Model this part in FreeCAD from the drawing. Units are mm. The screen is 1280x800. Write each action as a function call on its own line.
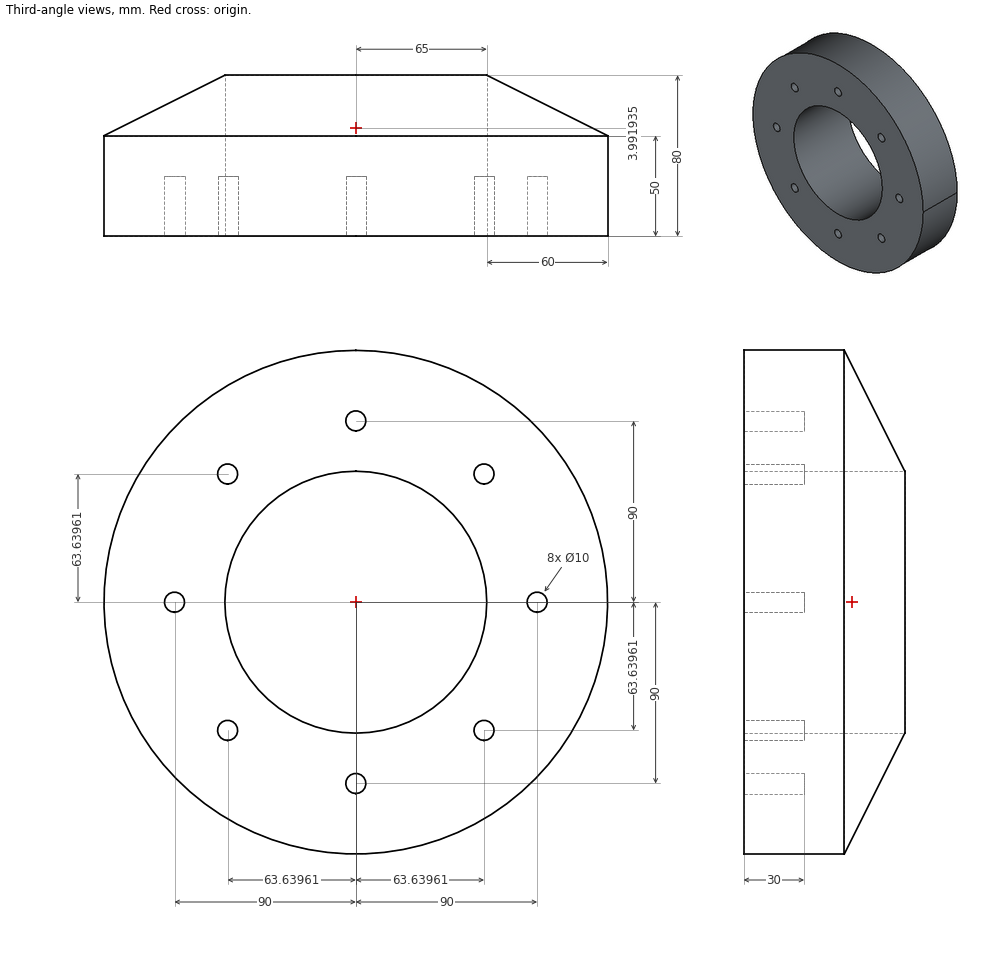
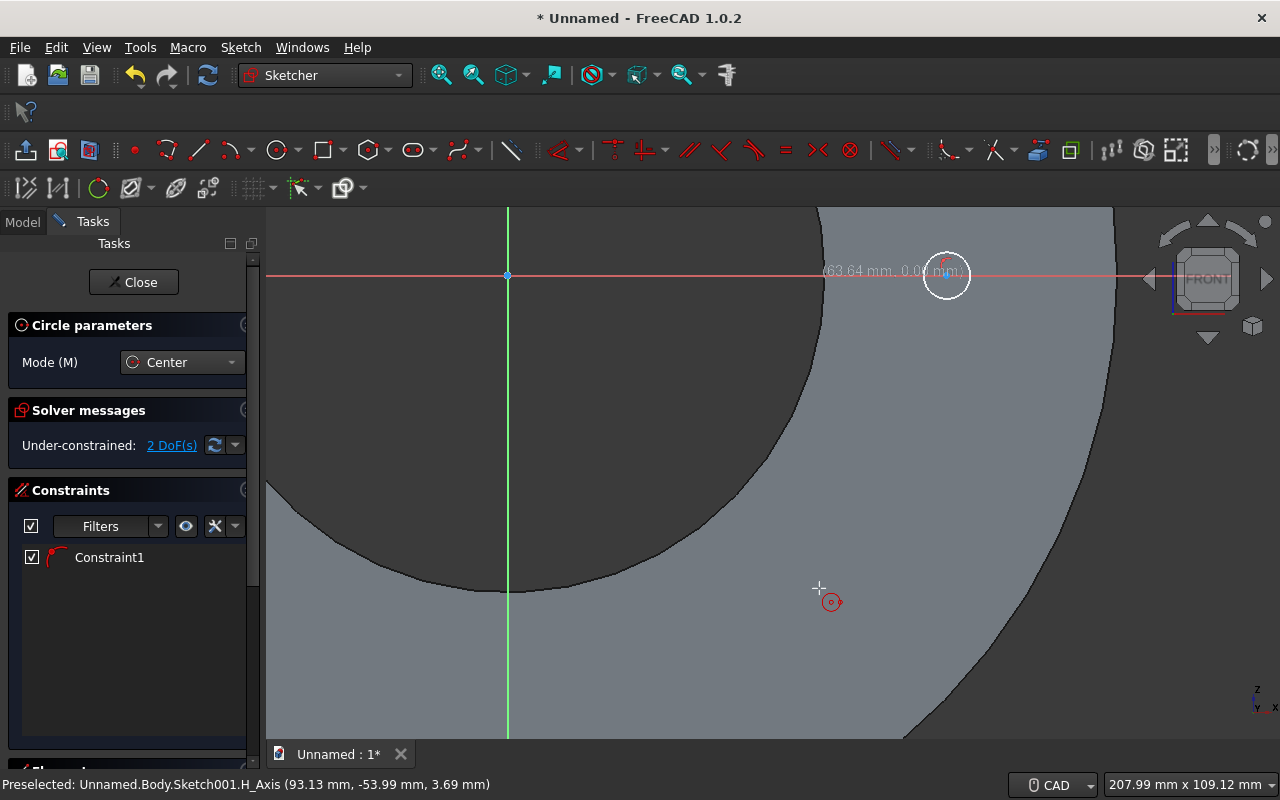
click(818, 586)
click(835, 569)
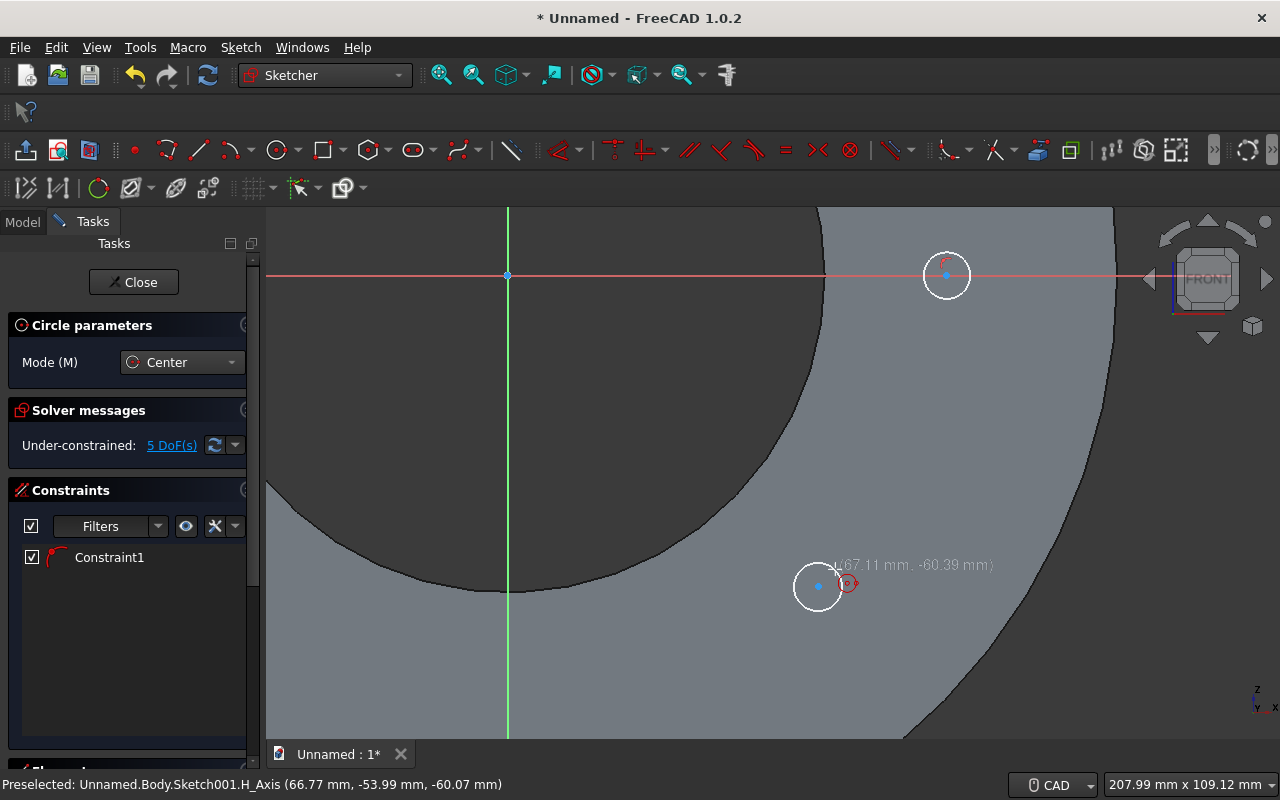
scroll(819, 588, down, 5)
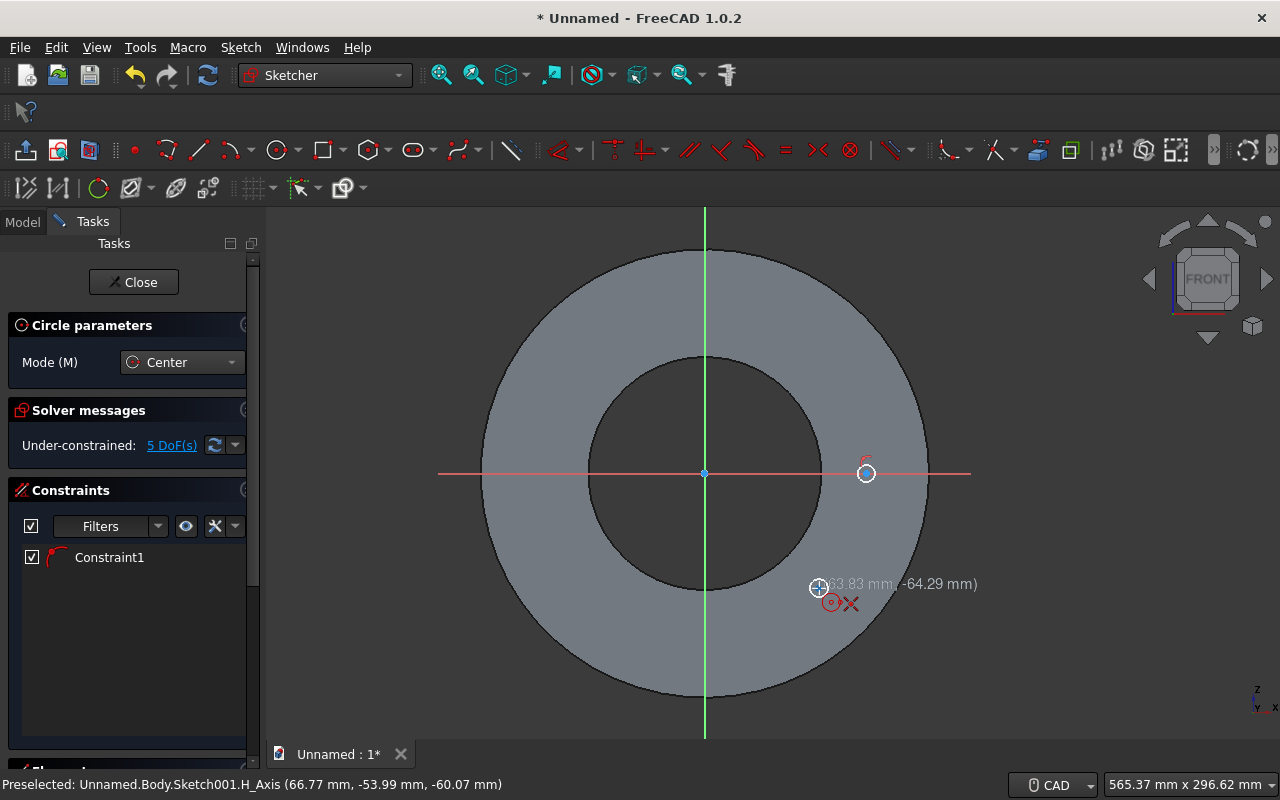
scroll(705, 635, up, 5)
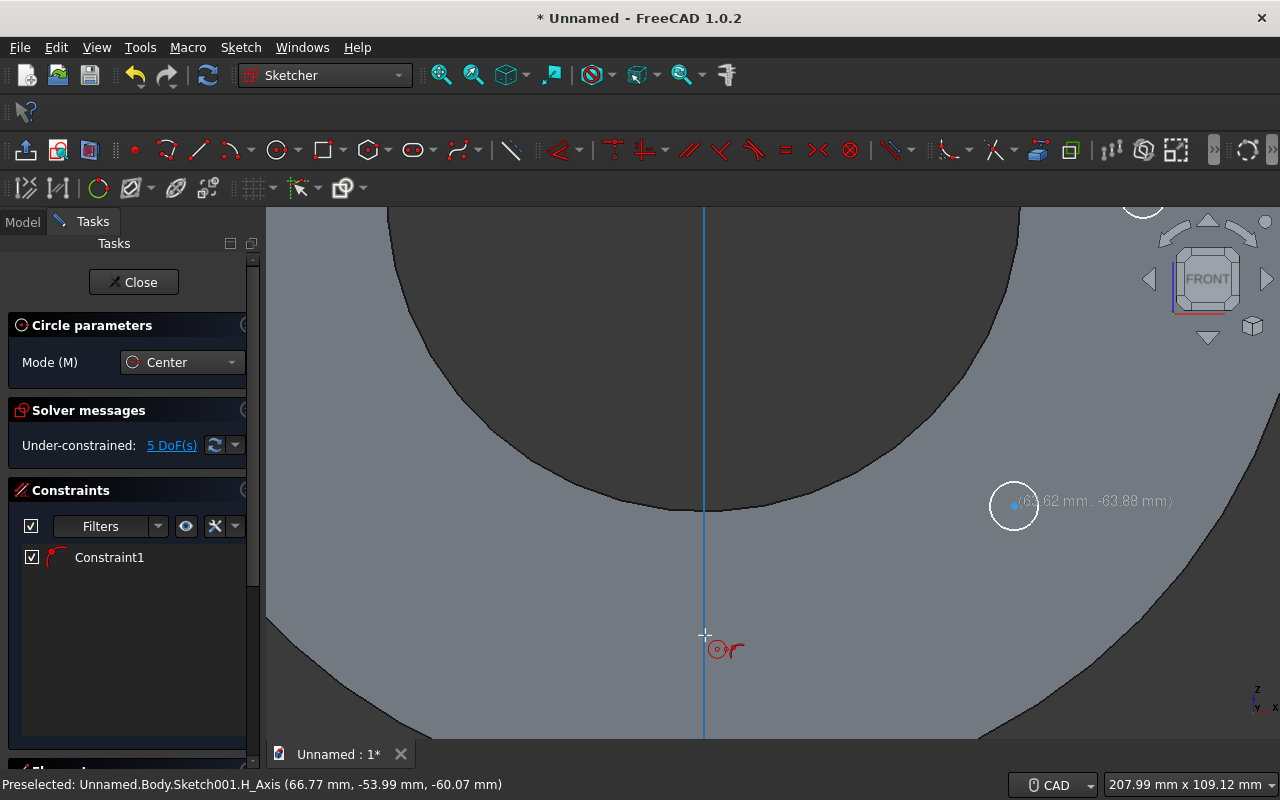
click(704, 633)
click(721, 616)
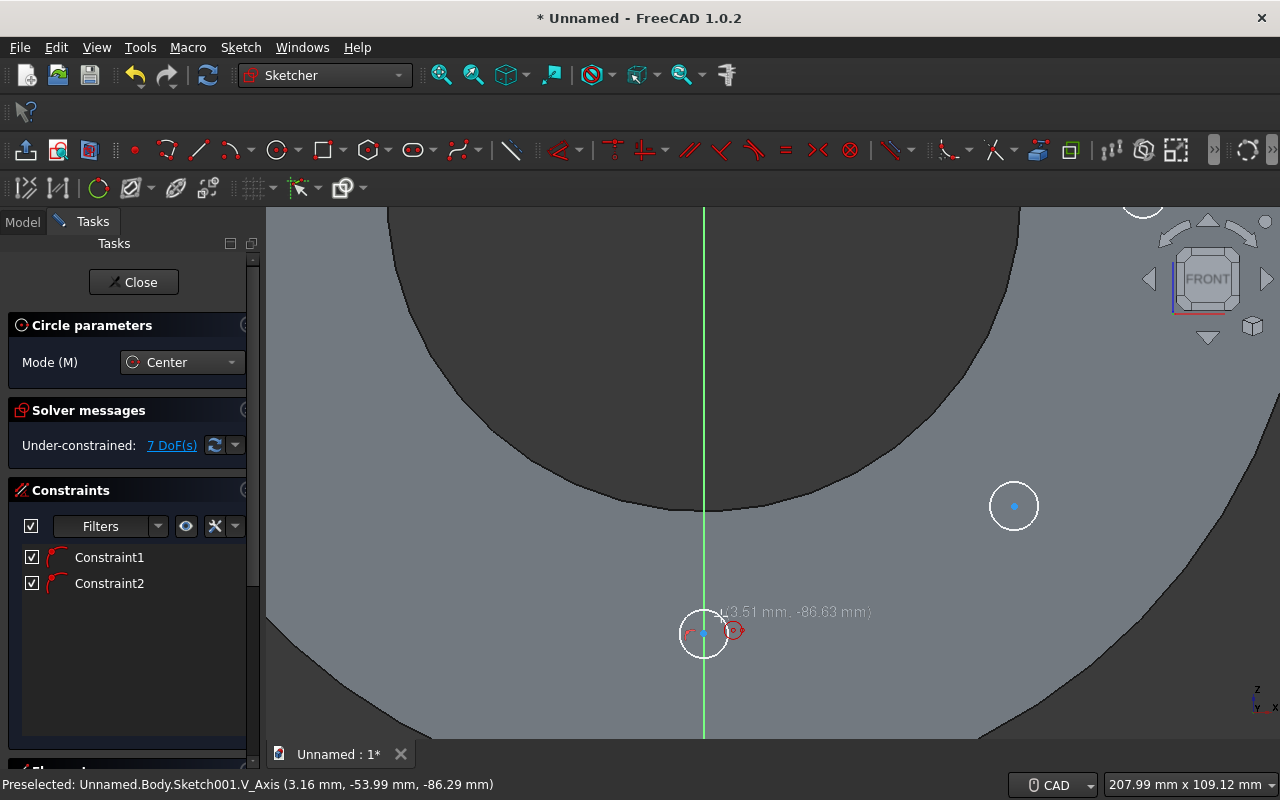
click(394, 505)
click(411, 488)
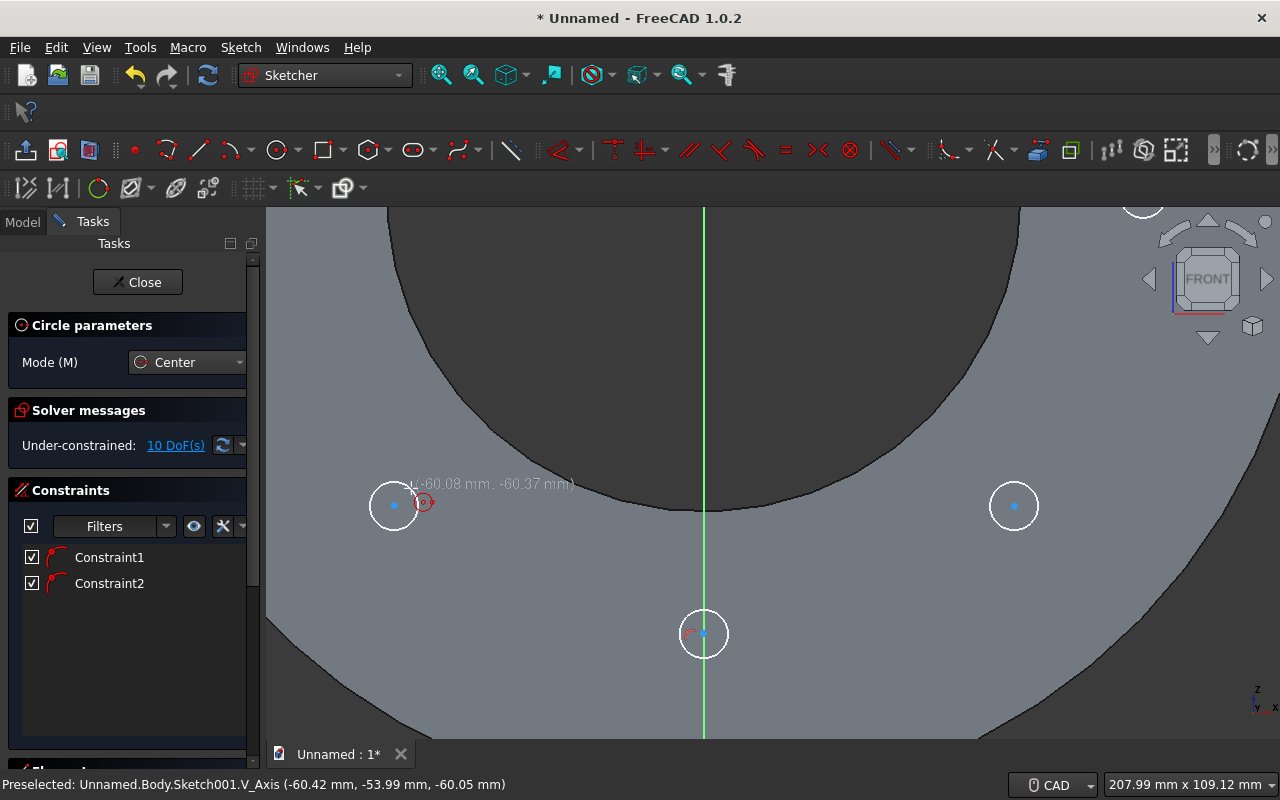
scroll(705, 635, down, 5)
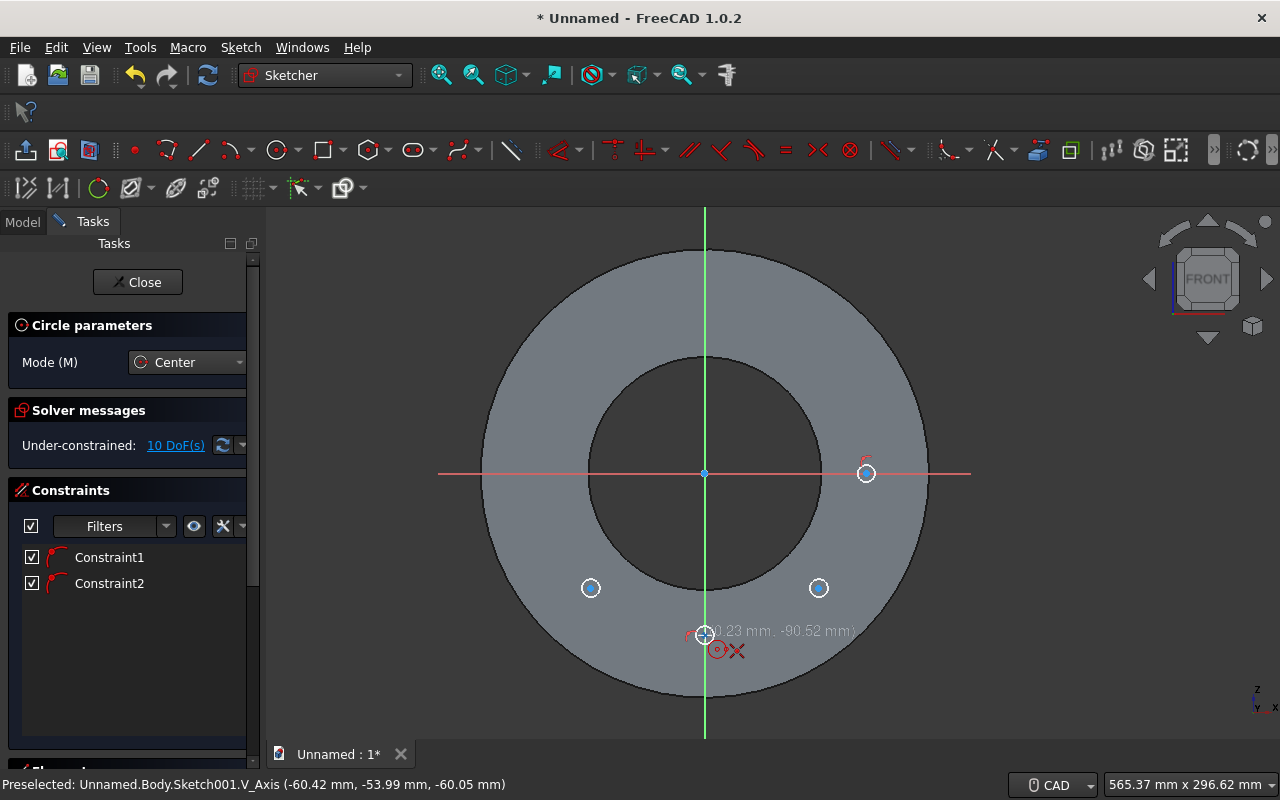
scroll(543, 474, up, 5)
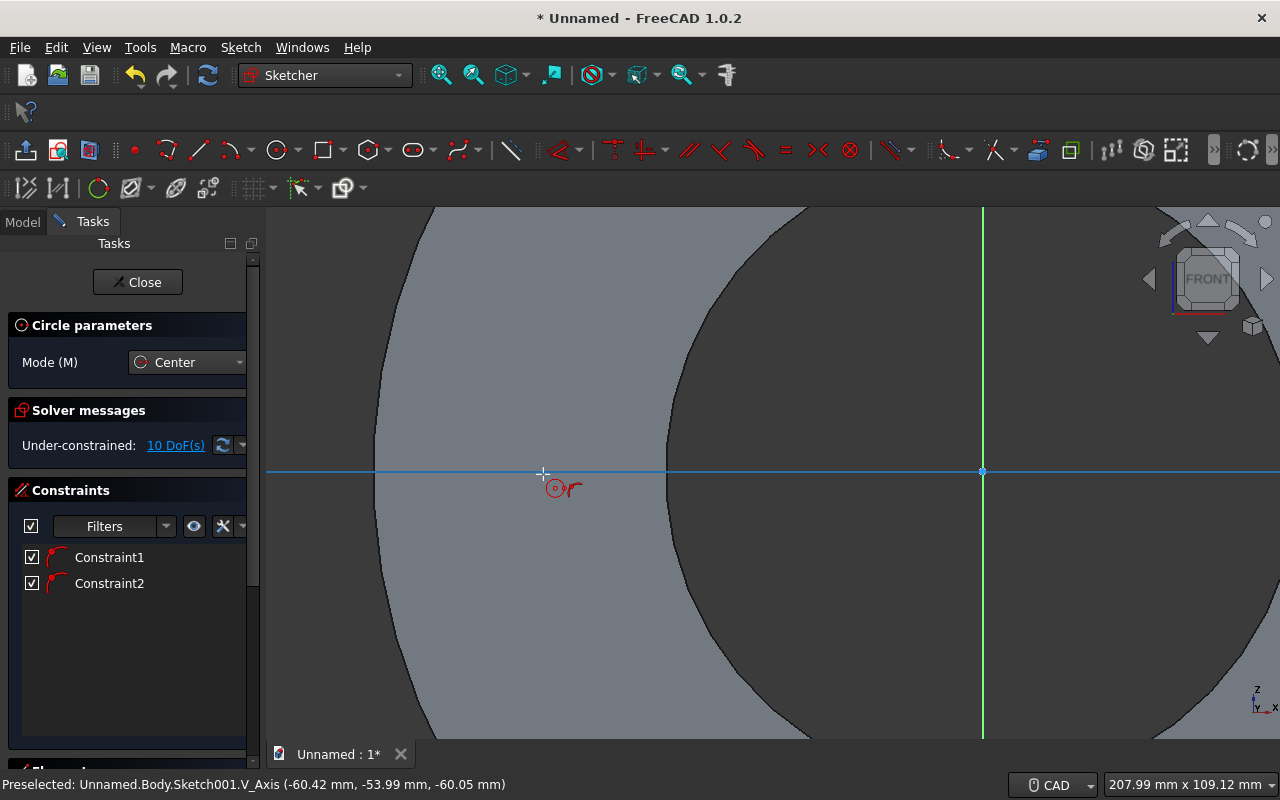
click(544, 472)
click(561, 455)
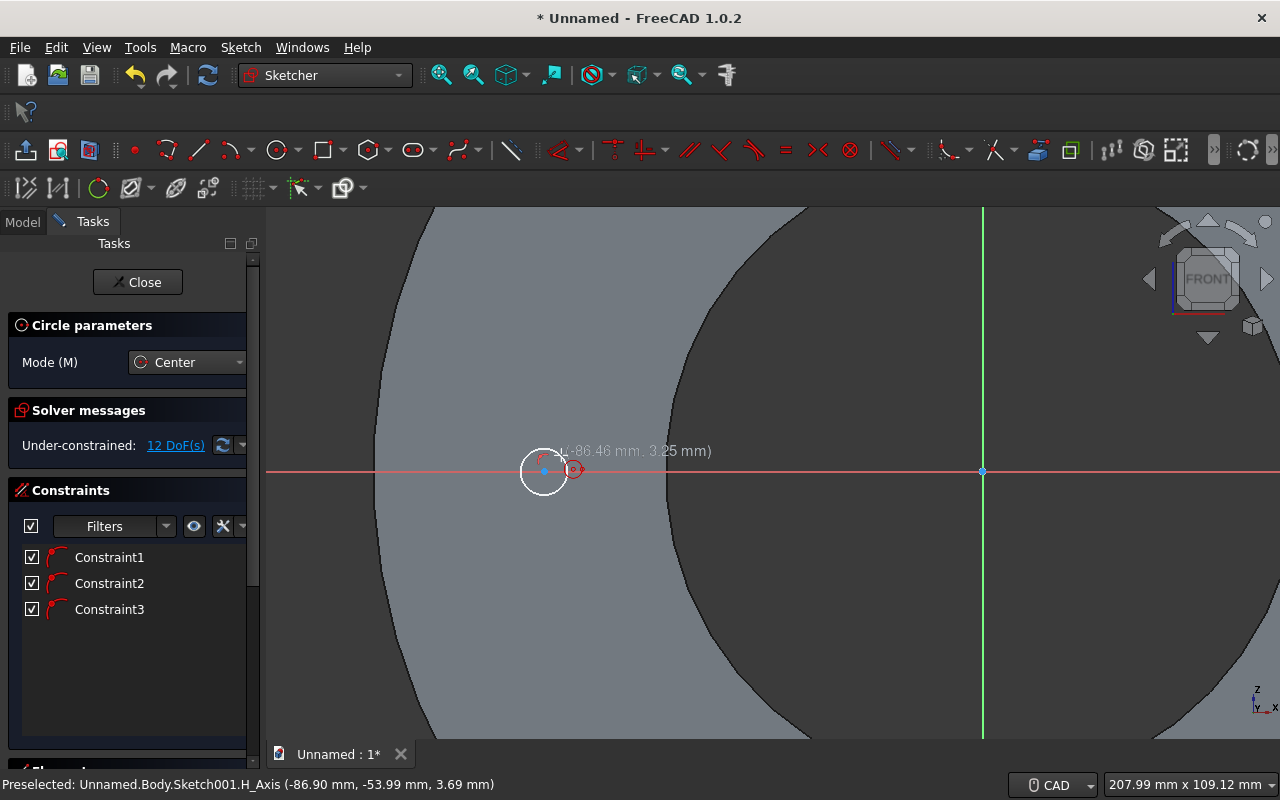
scroll(543, 474, down, 5)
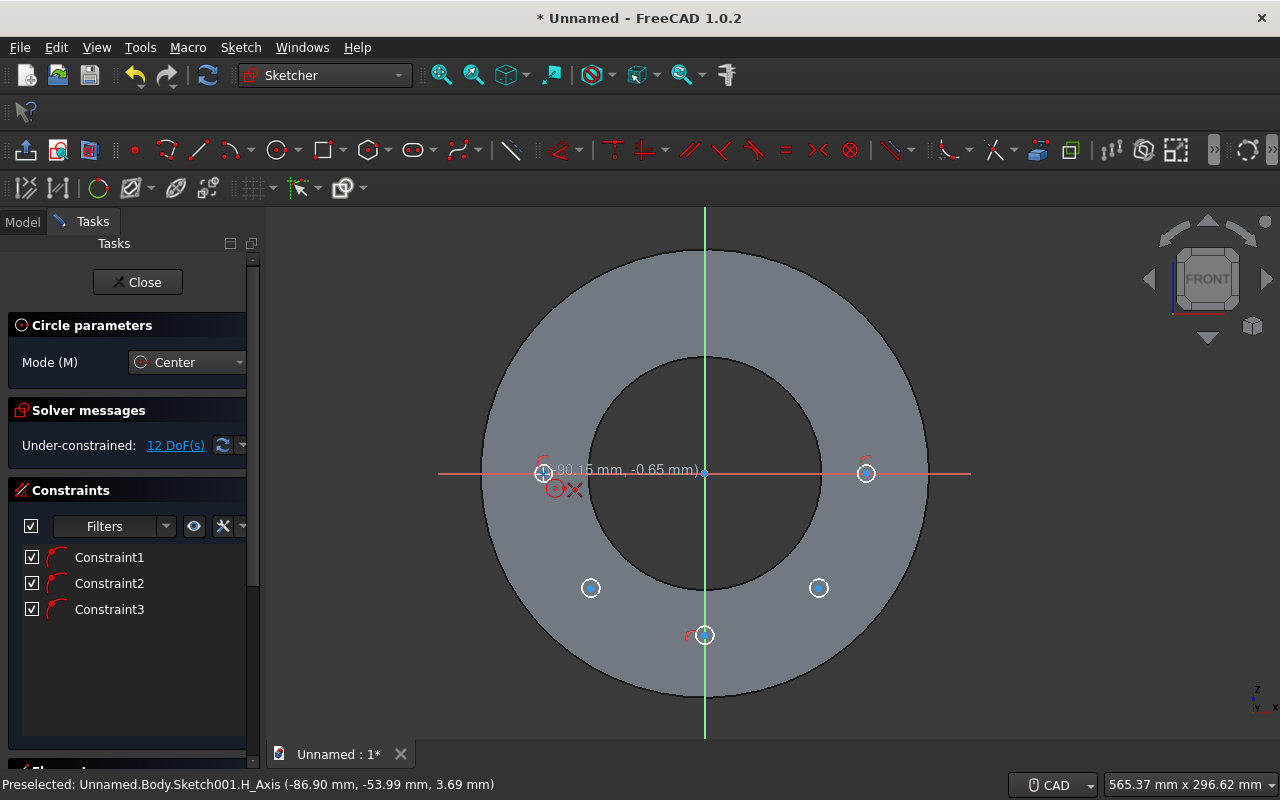
scroll(591, 359, up, 5)